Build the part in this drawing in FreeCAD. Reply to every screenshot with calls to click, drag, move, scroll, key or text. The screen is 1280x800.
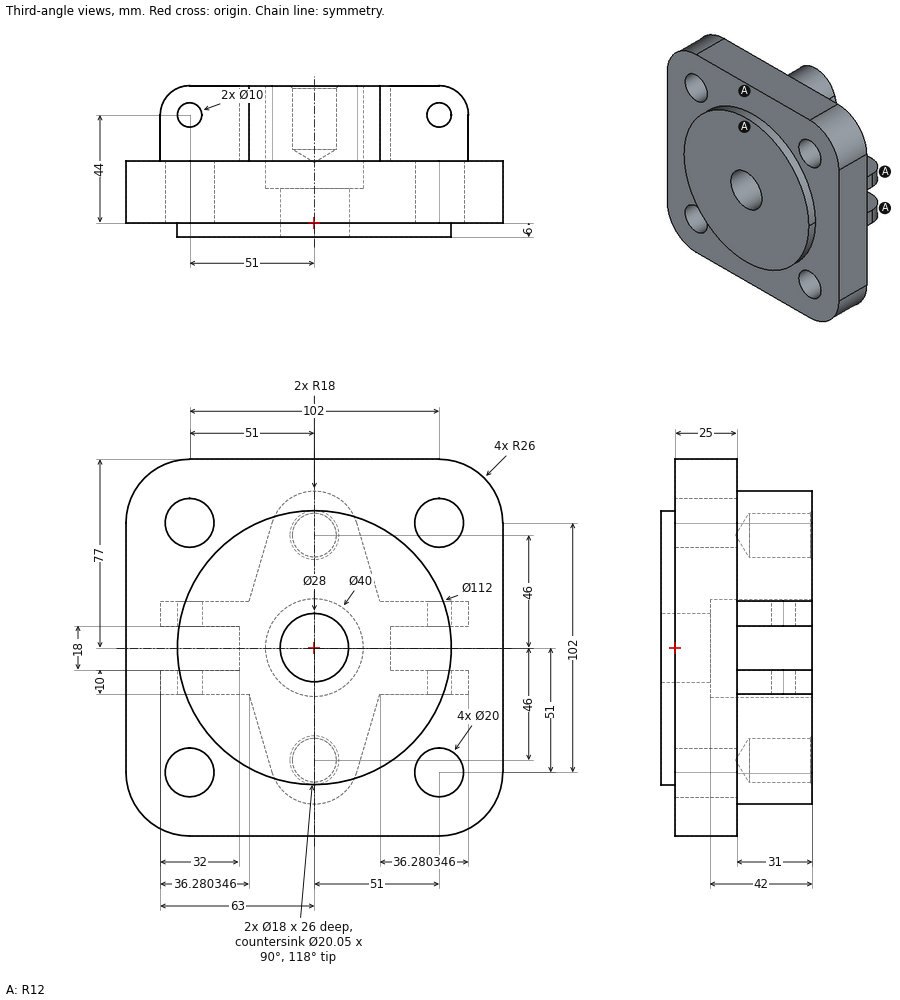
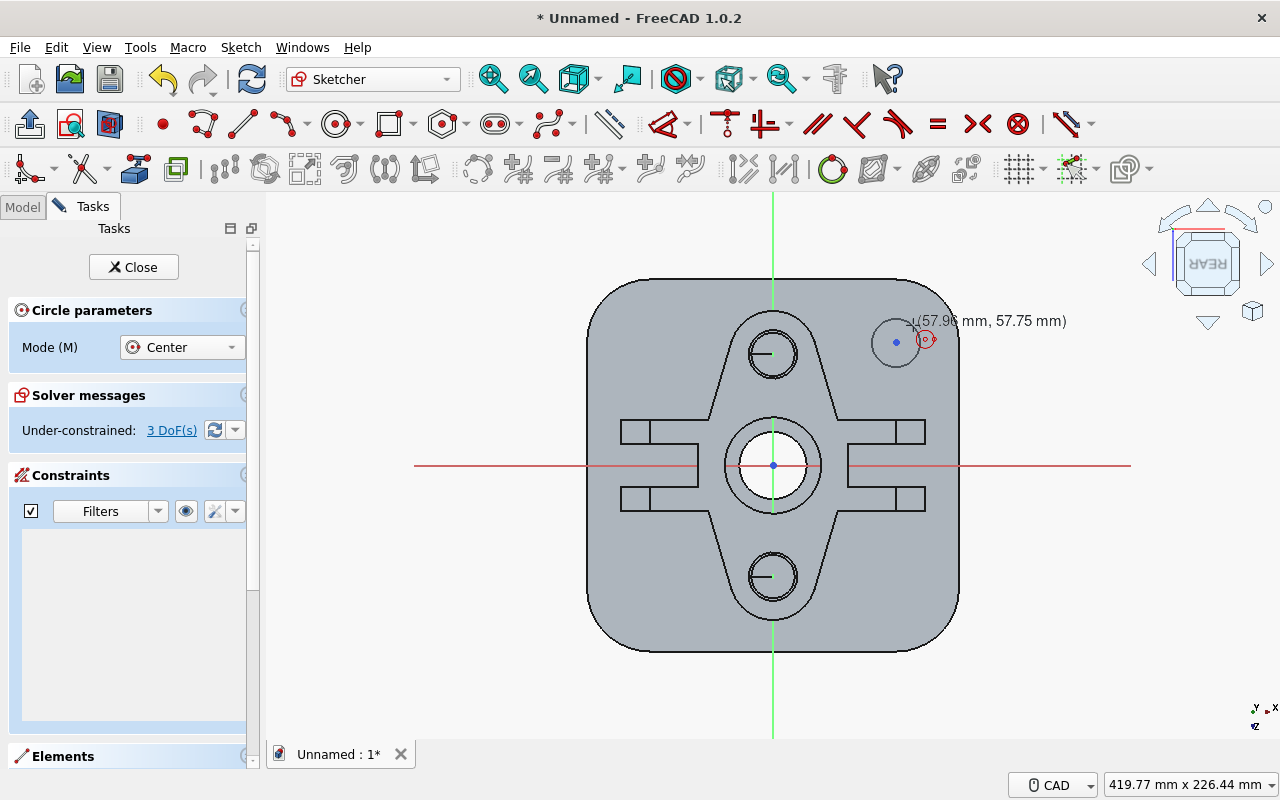
click(650, 342)
click(667, 325)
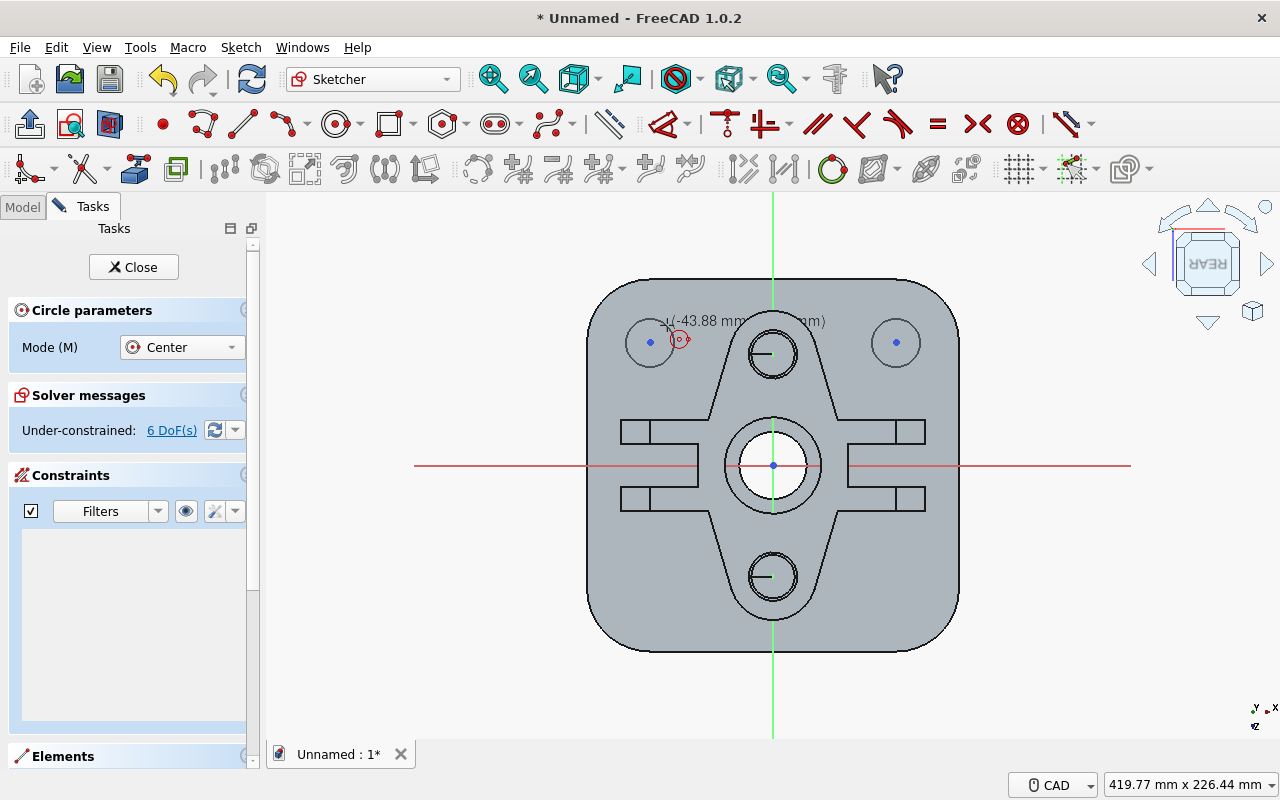
click(650, 589)
click(667, 572)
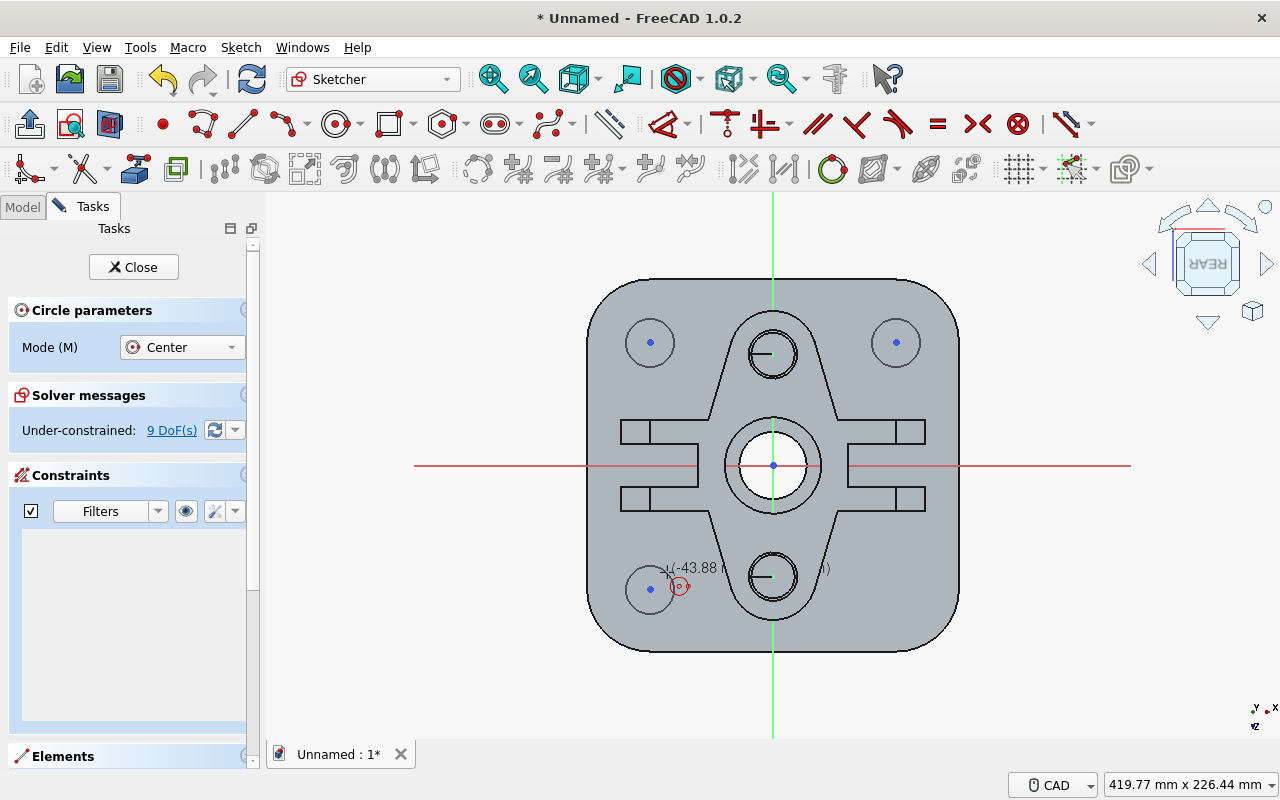
click(896, 589)
click(913, 572)
key(Escape)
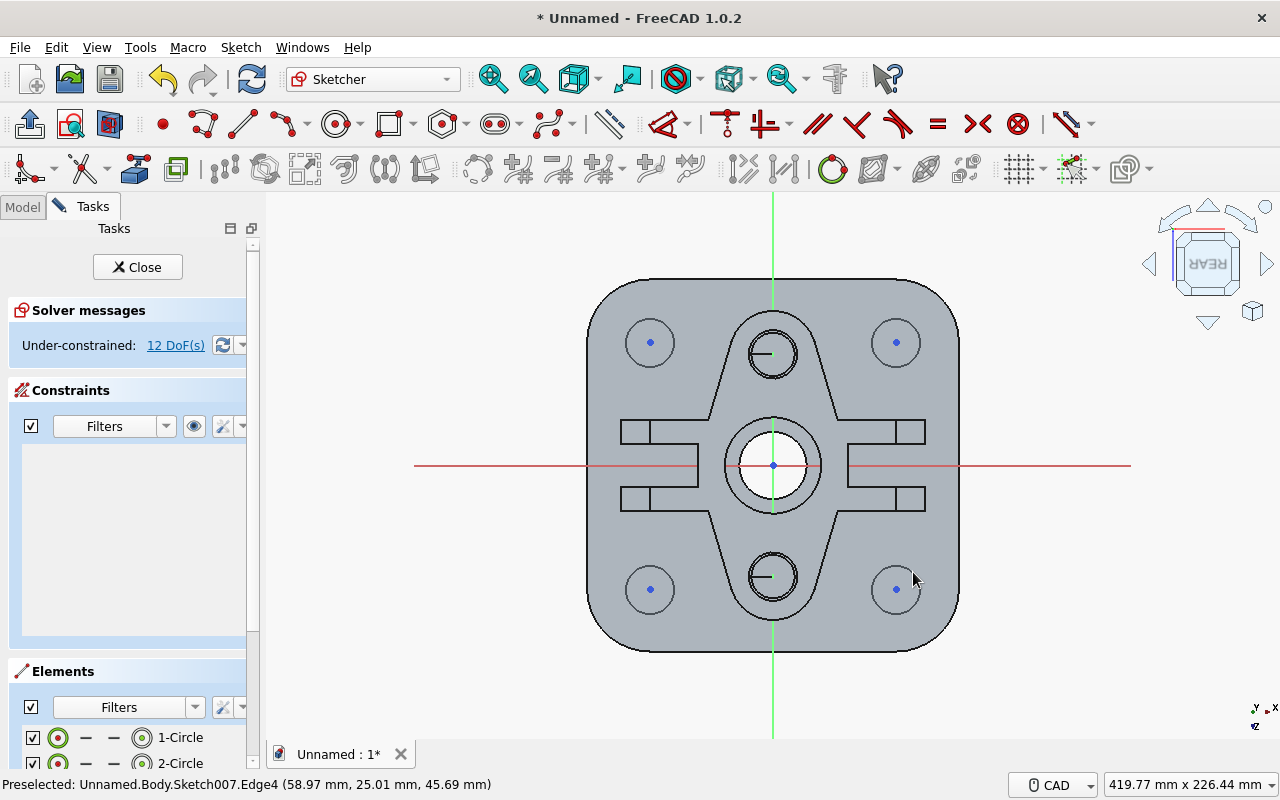
click(913, 326)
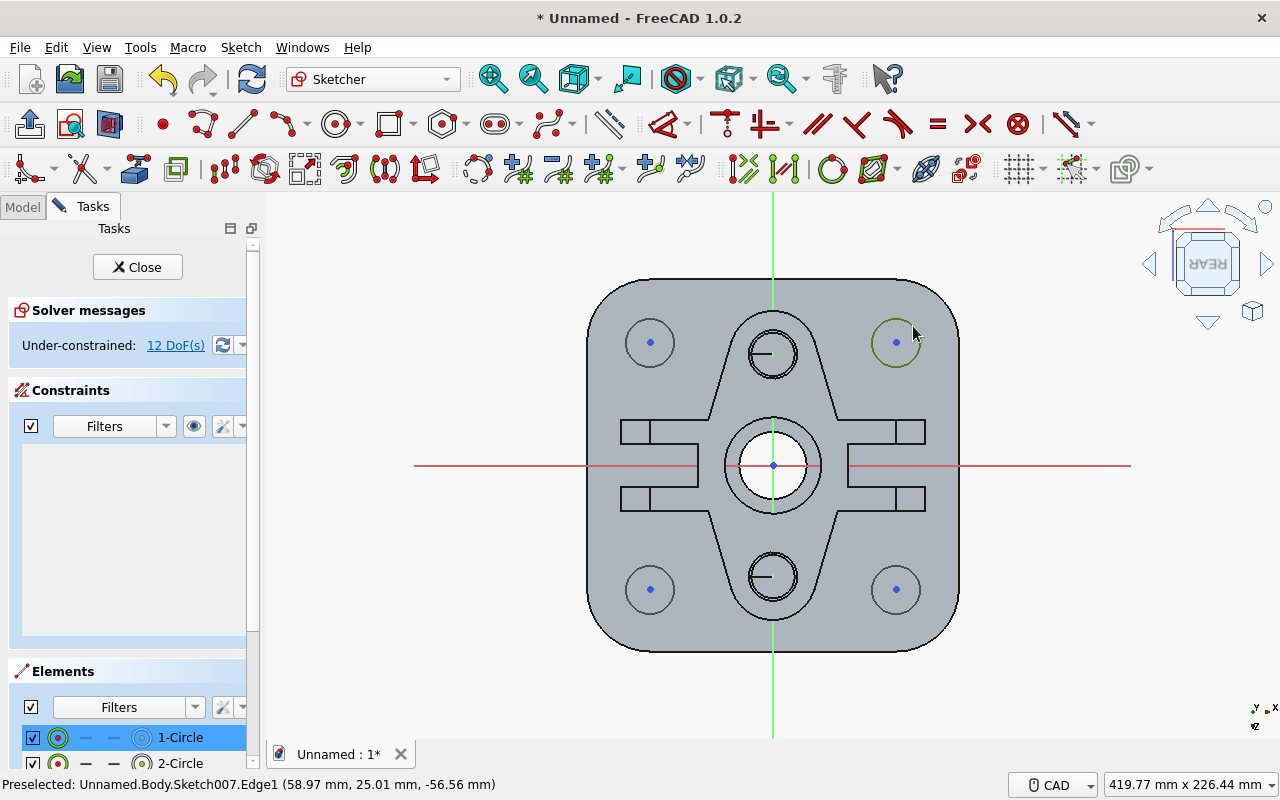
click(667, 326)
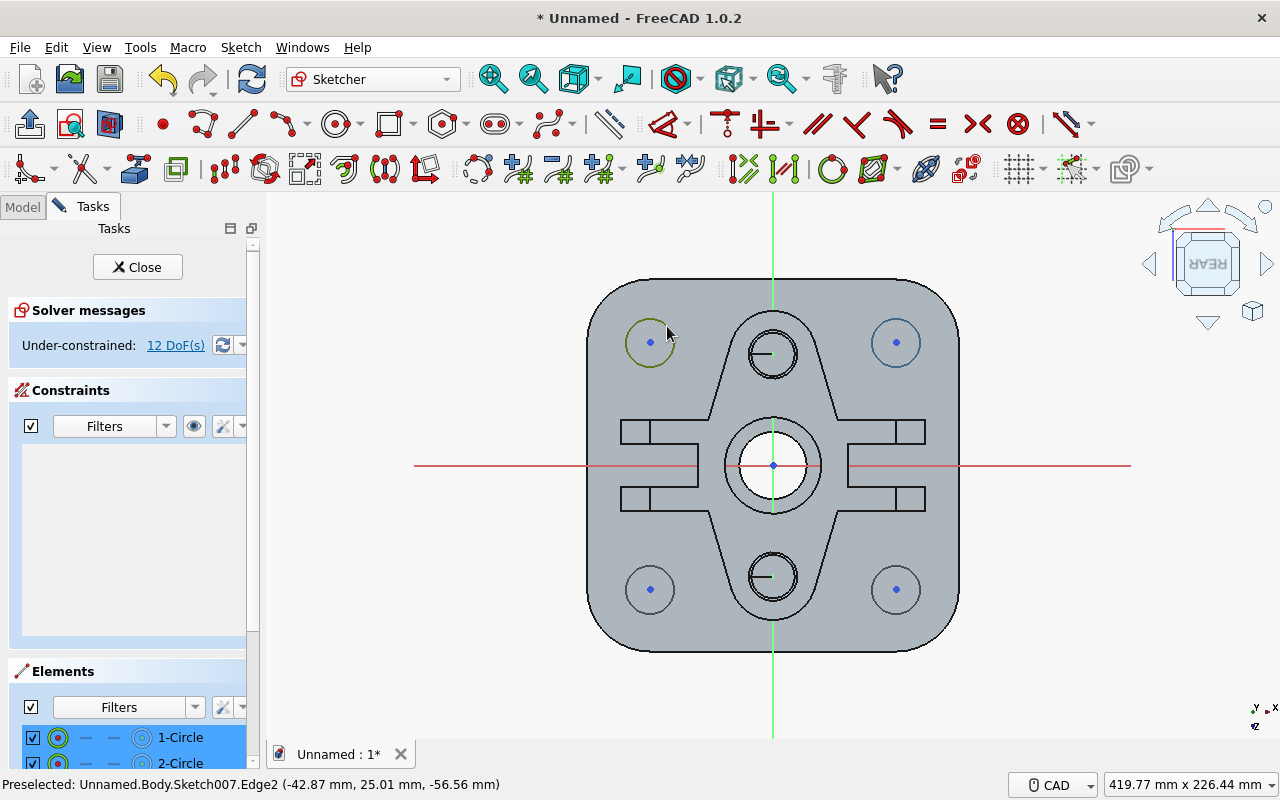
click(667, 573)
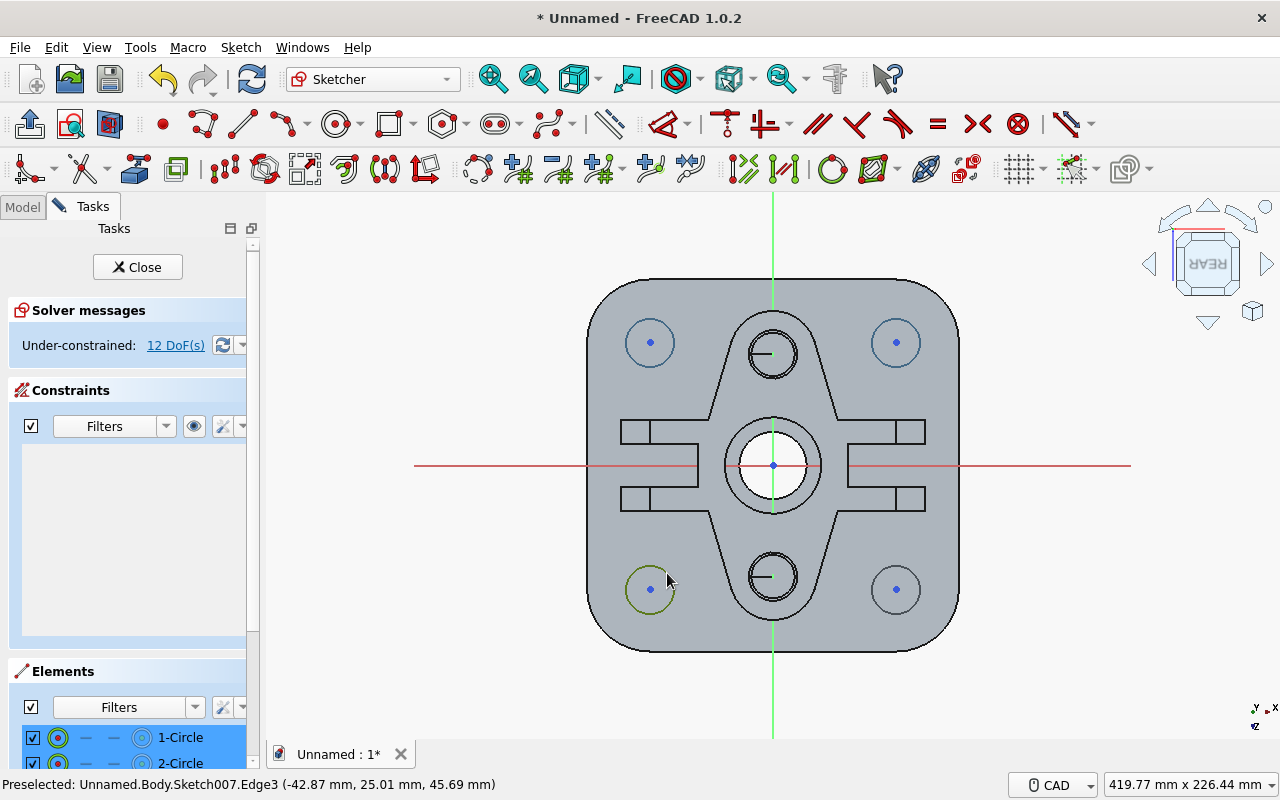
click(913, 573)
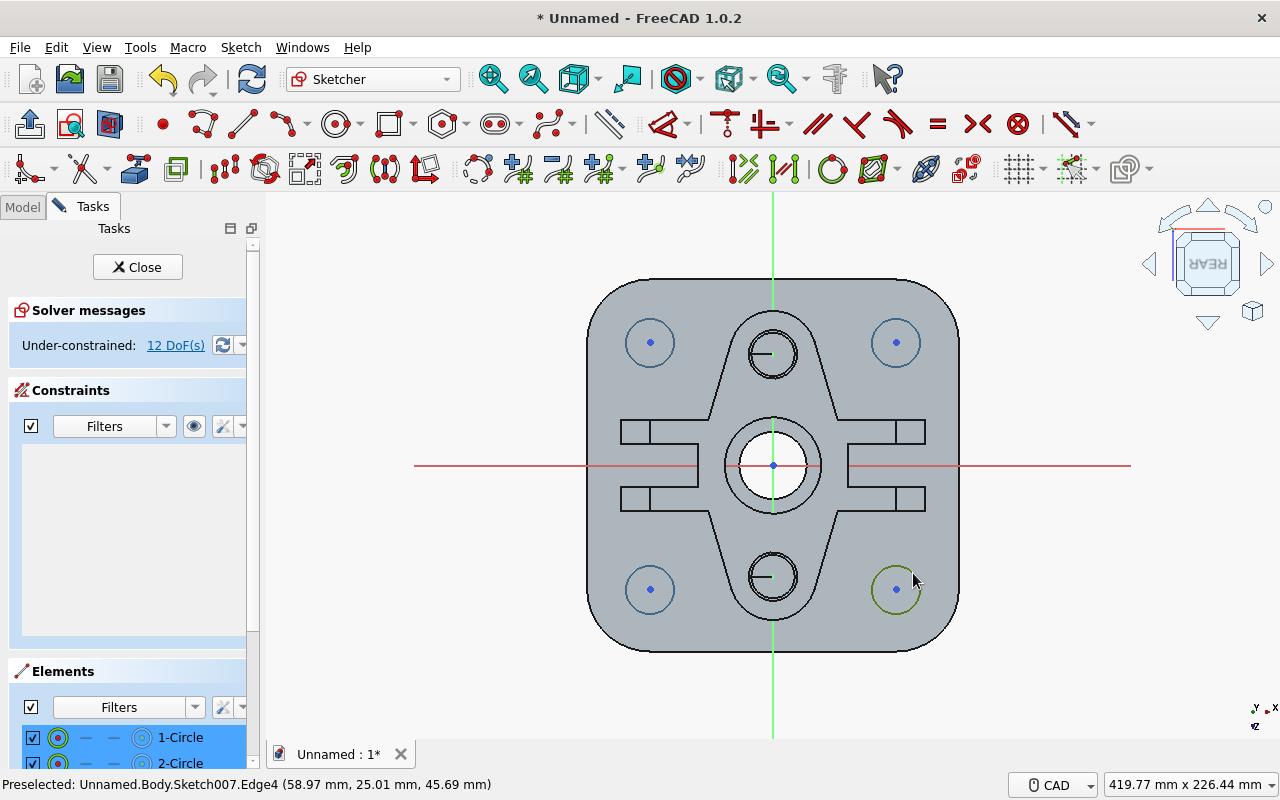
key(e)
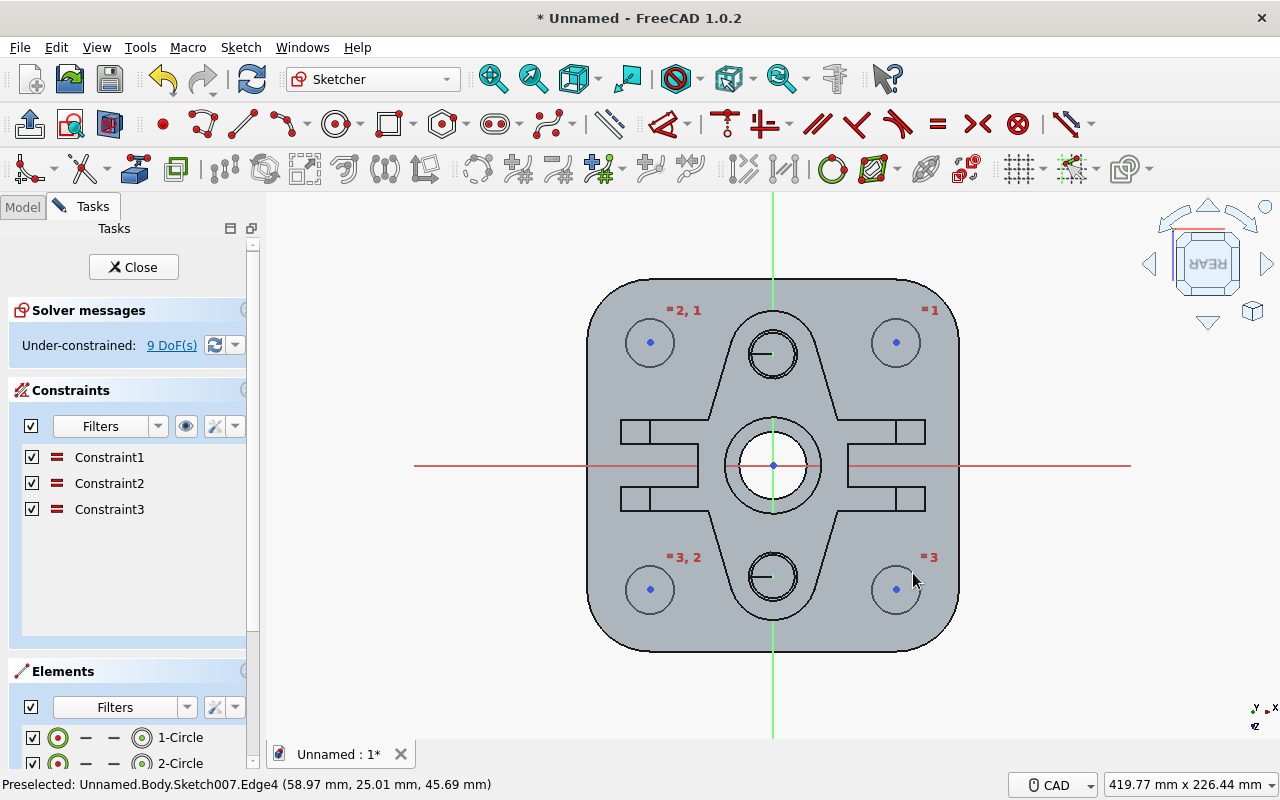
click(896, 343)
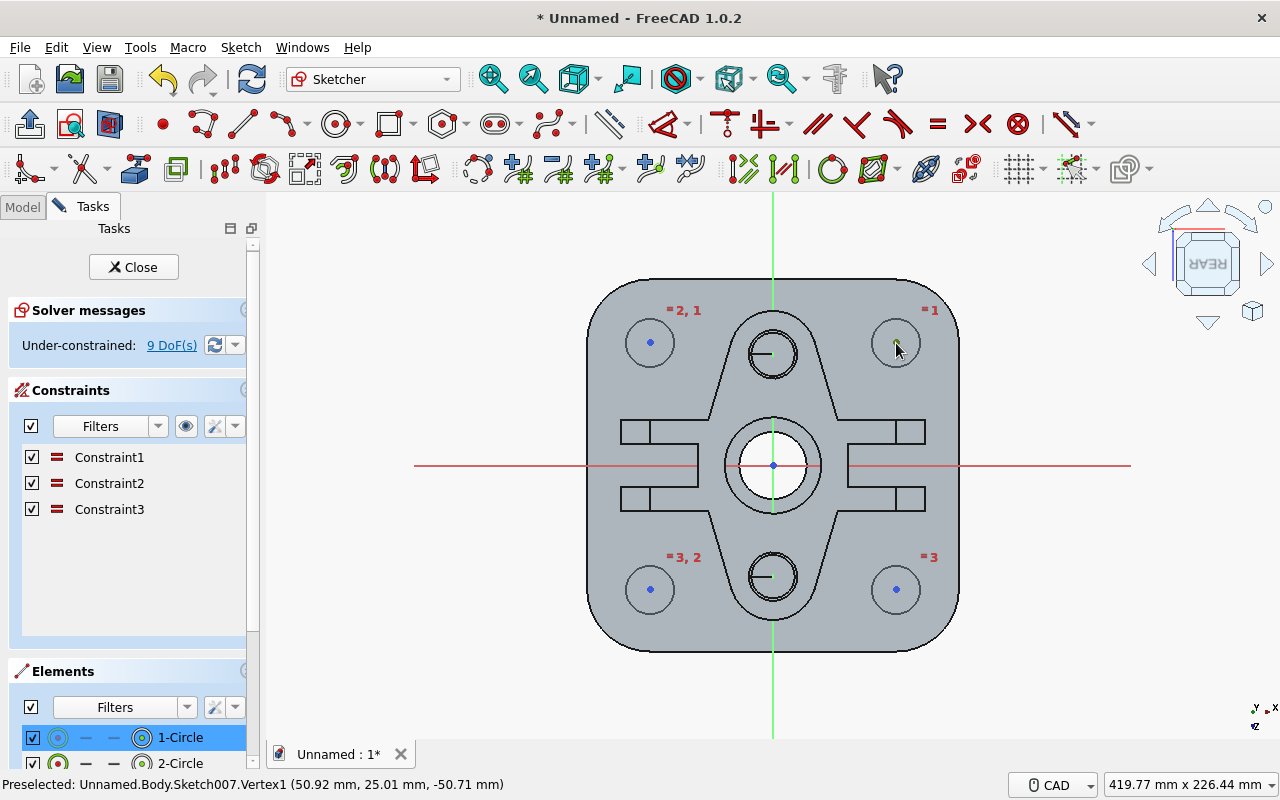
click(650, 343)